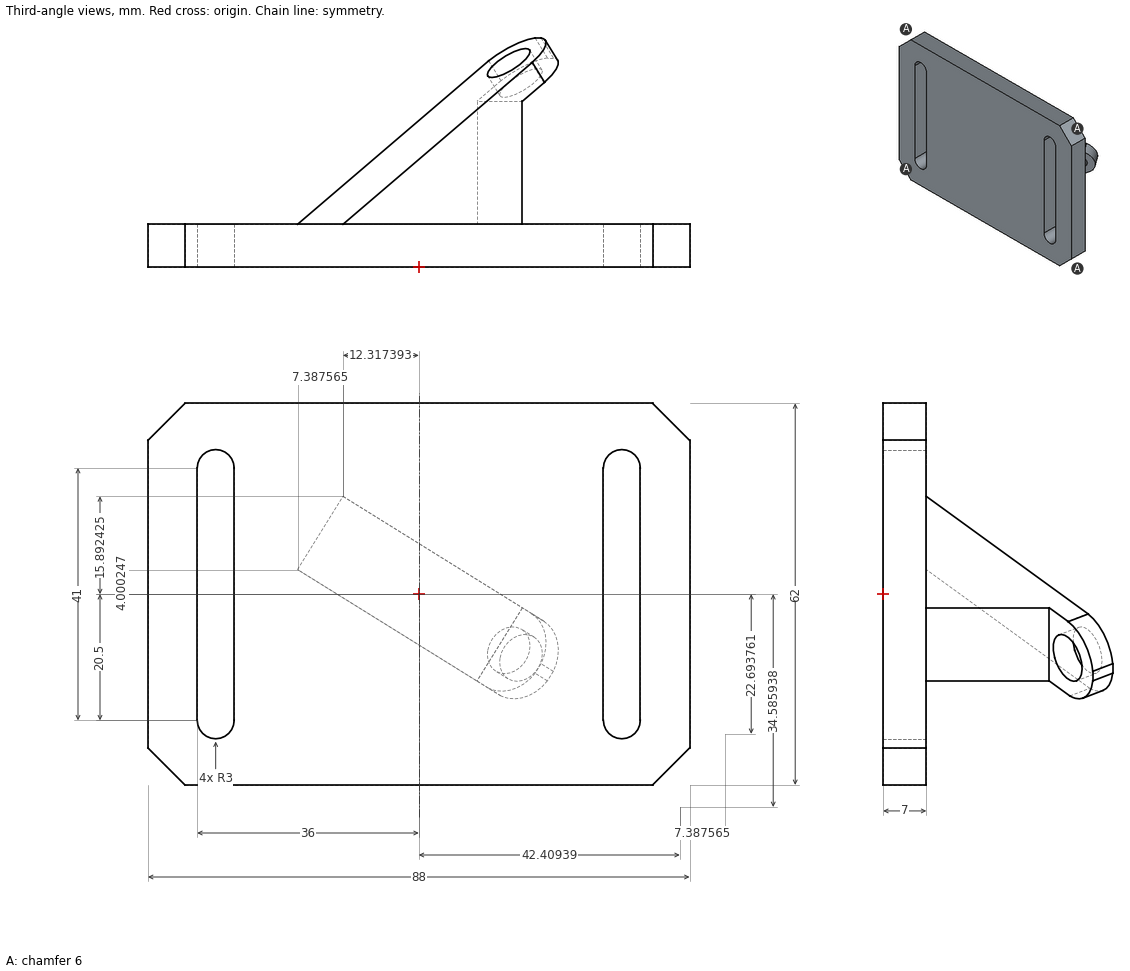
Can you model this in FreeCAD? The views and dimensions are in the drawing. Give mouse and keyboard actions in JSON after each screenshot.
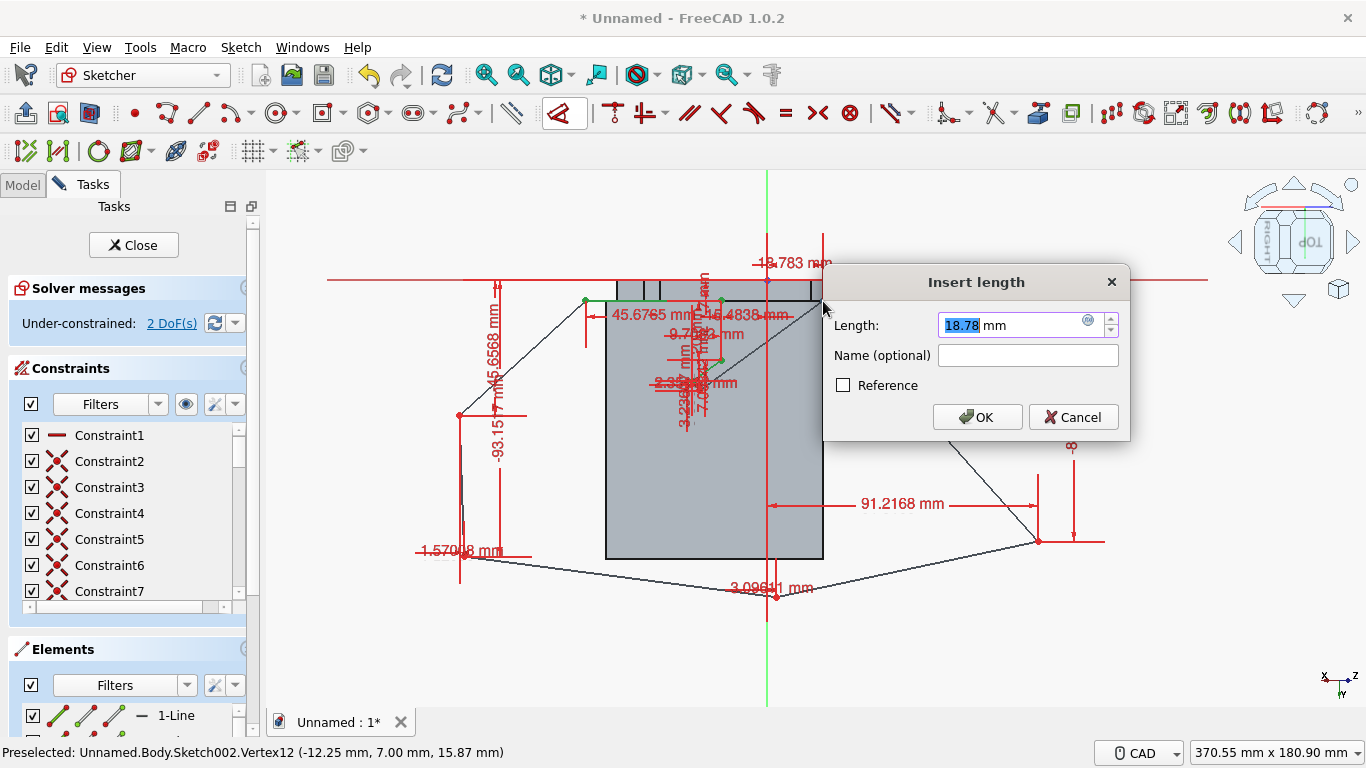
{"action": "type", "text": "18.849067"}
{"action": "key", "text": "Return"}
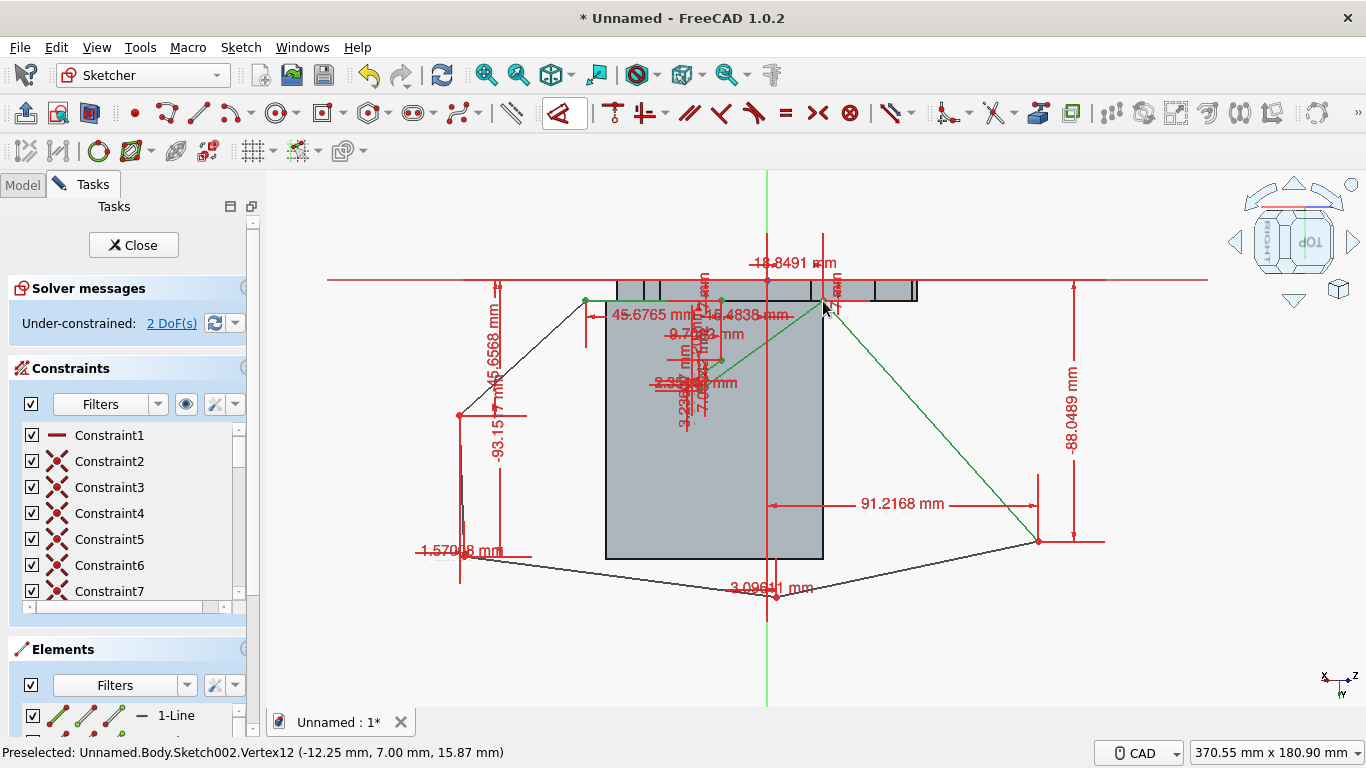
{"action": "left_click", "coordinate": [548, 335]}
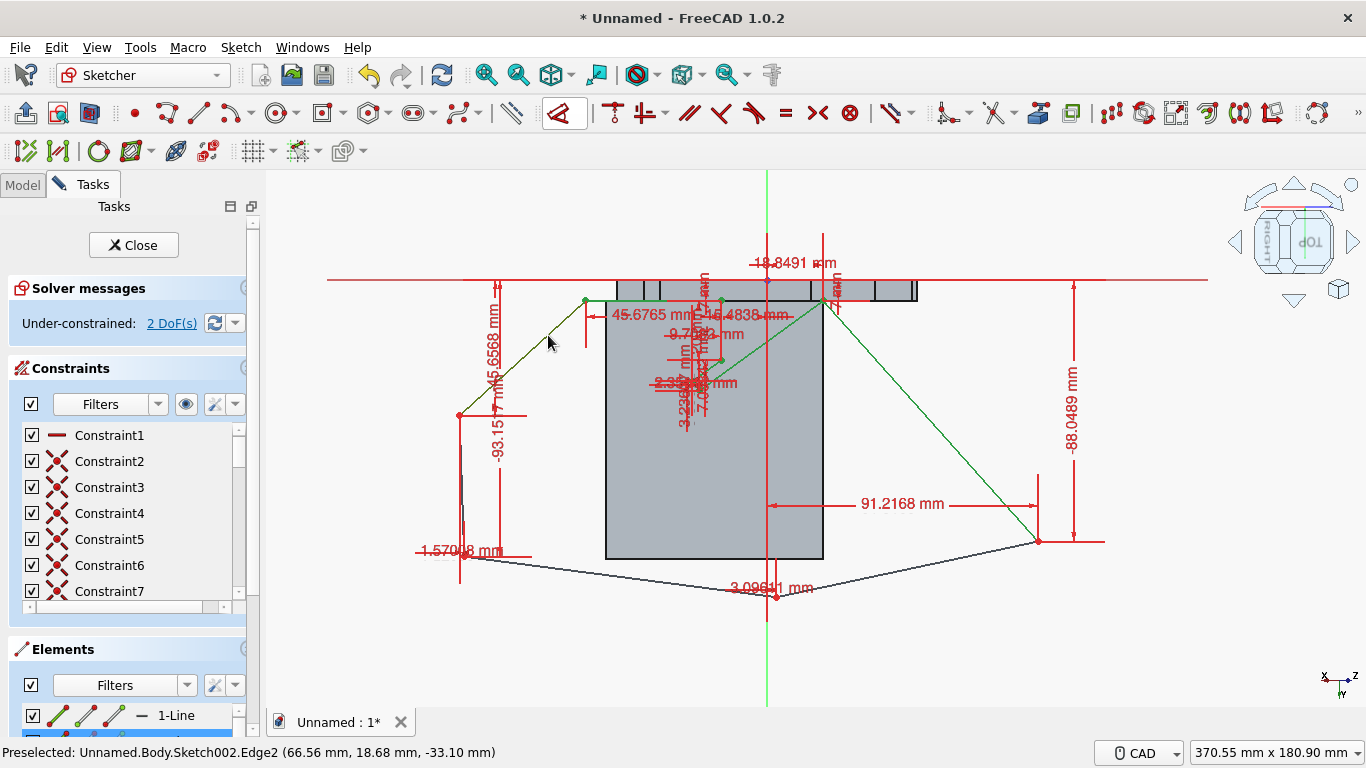
{"action": "key", "text": "l"}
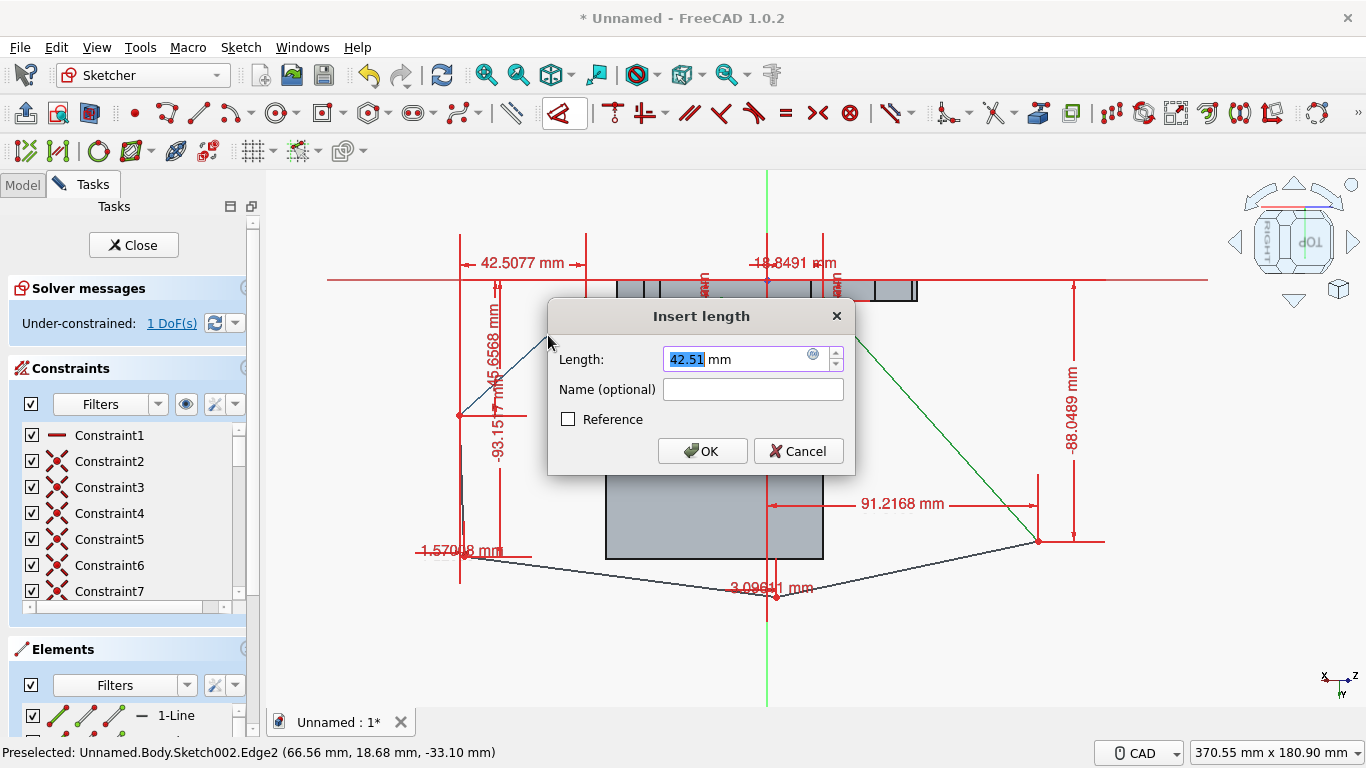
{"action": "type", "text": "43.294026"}
{"action": "key", "text": "Return"}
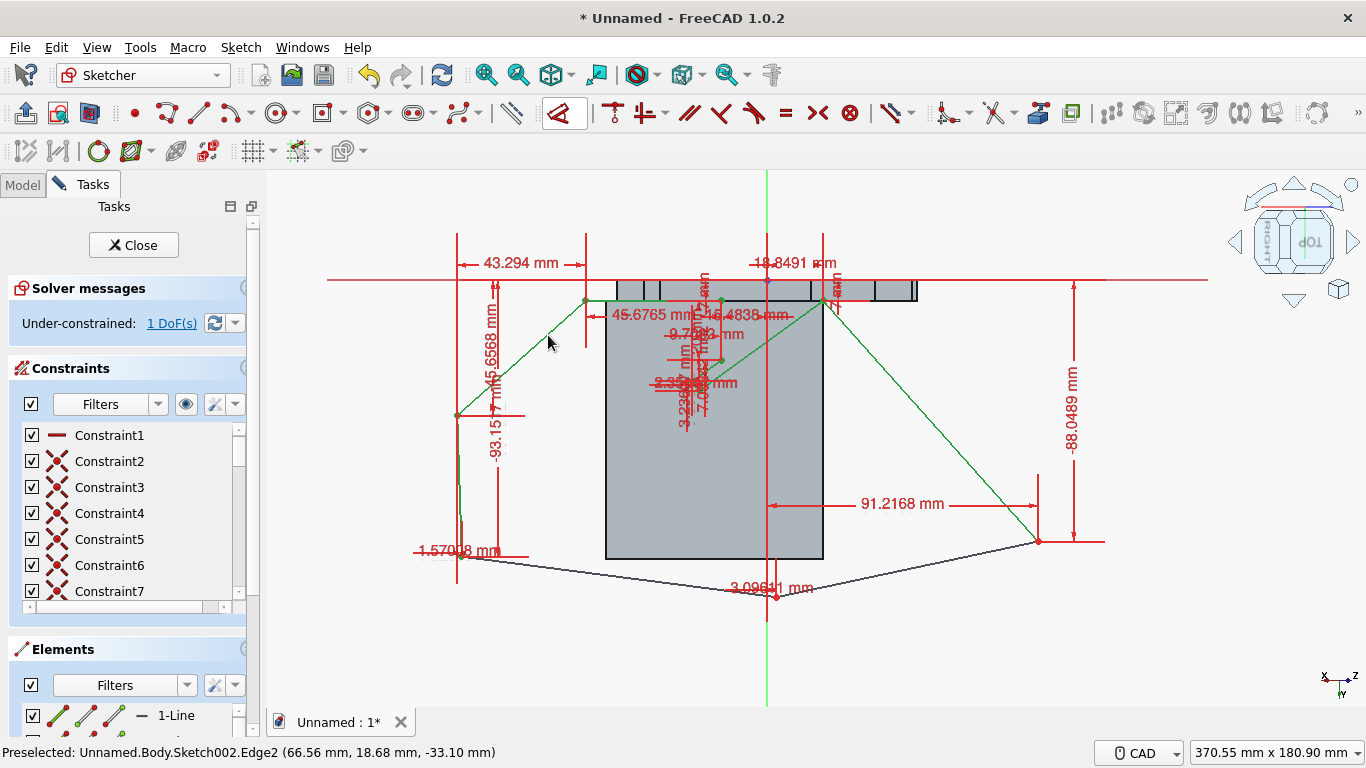
{"action": "left_click", "coordinate": [556, 569]}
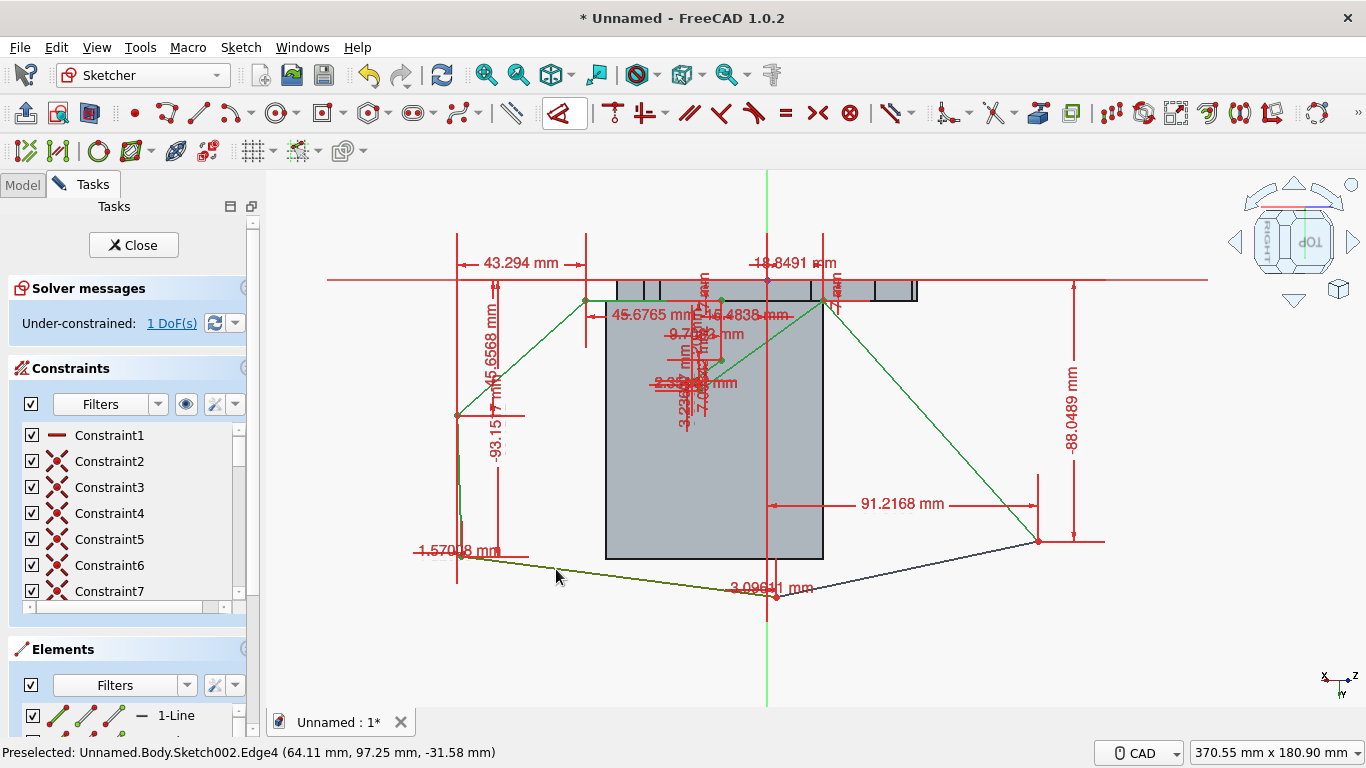
{"action": "left_click", "coordinate": [582, 114]}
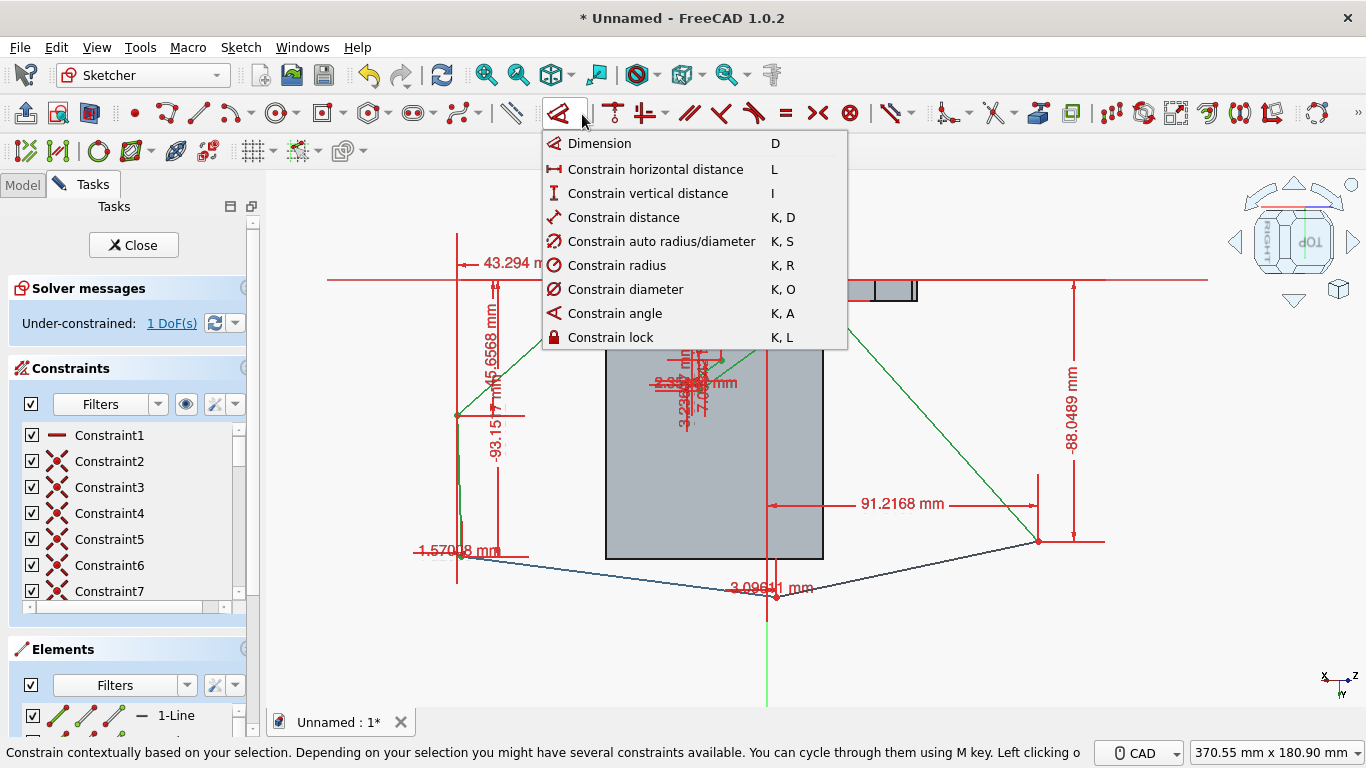
{"action": "left_click", "coordinate": [695, 193]}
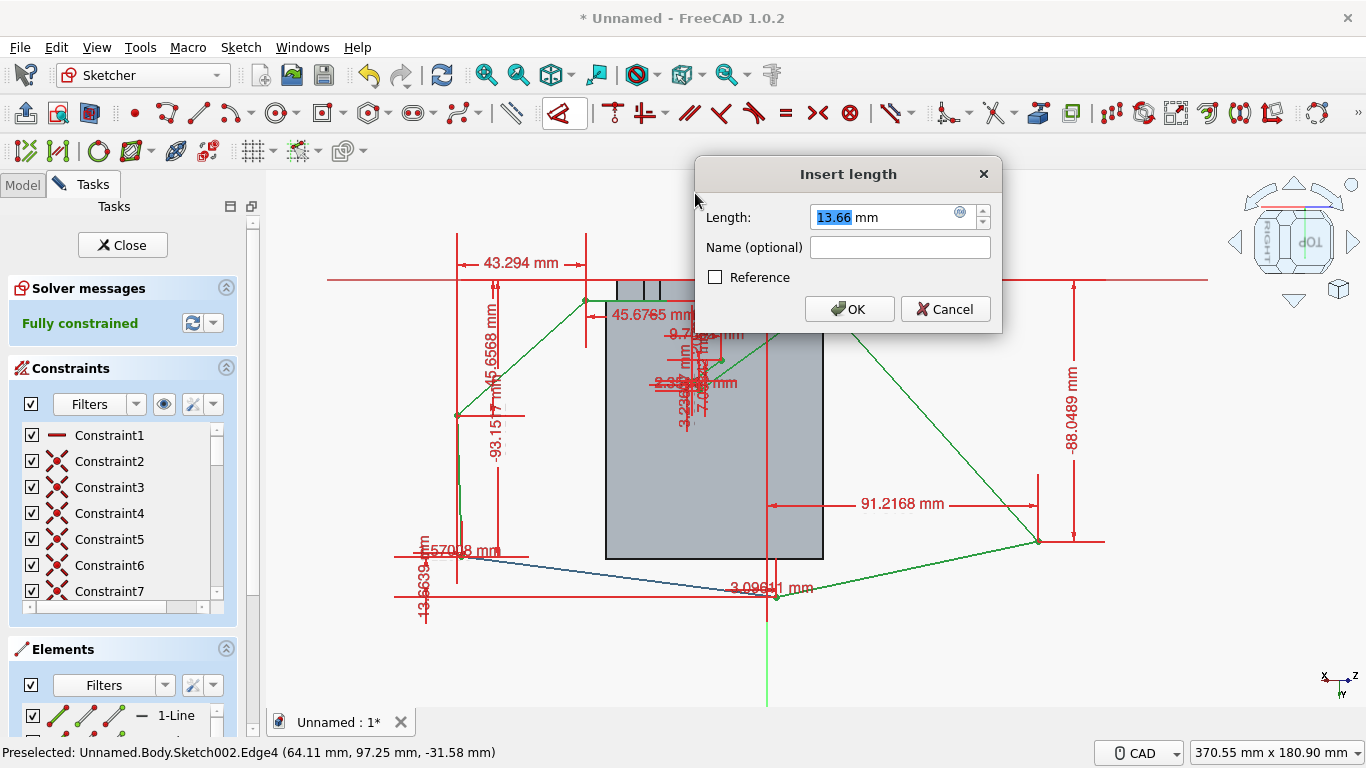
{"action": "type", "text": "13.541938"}
{"action": "key", "text": "Return"}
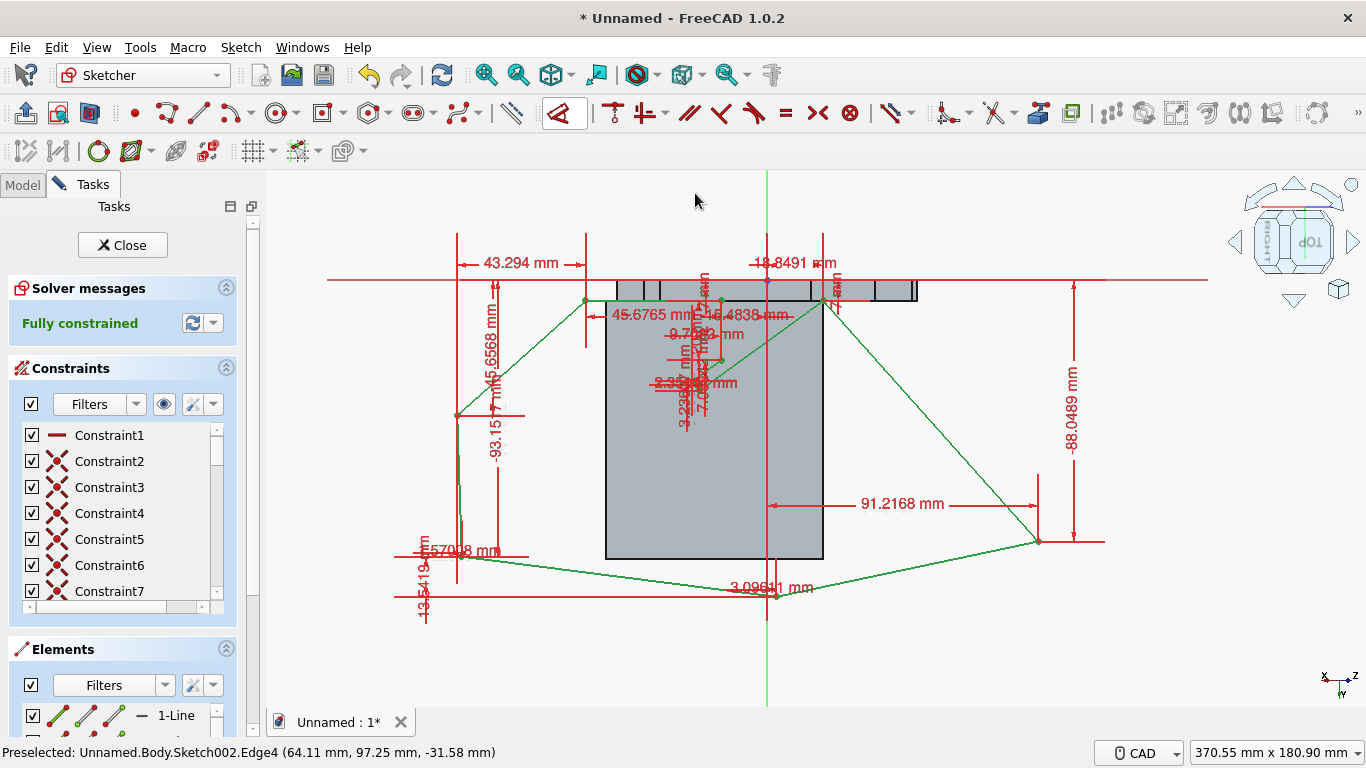
{"action": "left_click", "coordinate": [123, 245]}